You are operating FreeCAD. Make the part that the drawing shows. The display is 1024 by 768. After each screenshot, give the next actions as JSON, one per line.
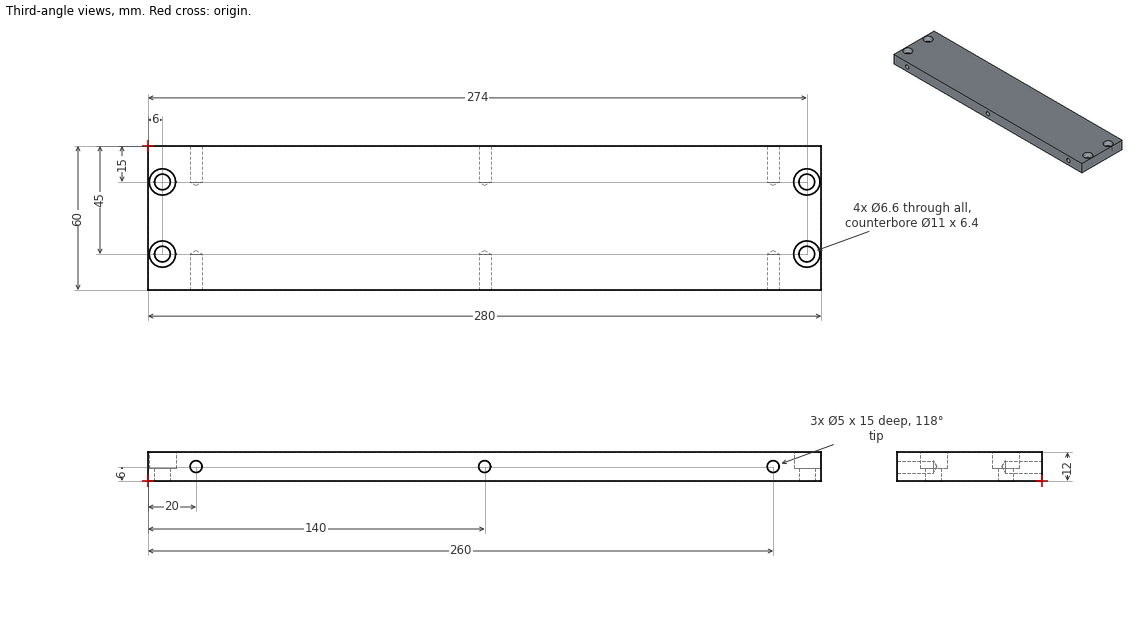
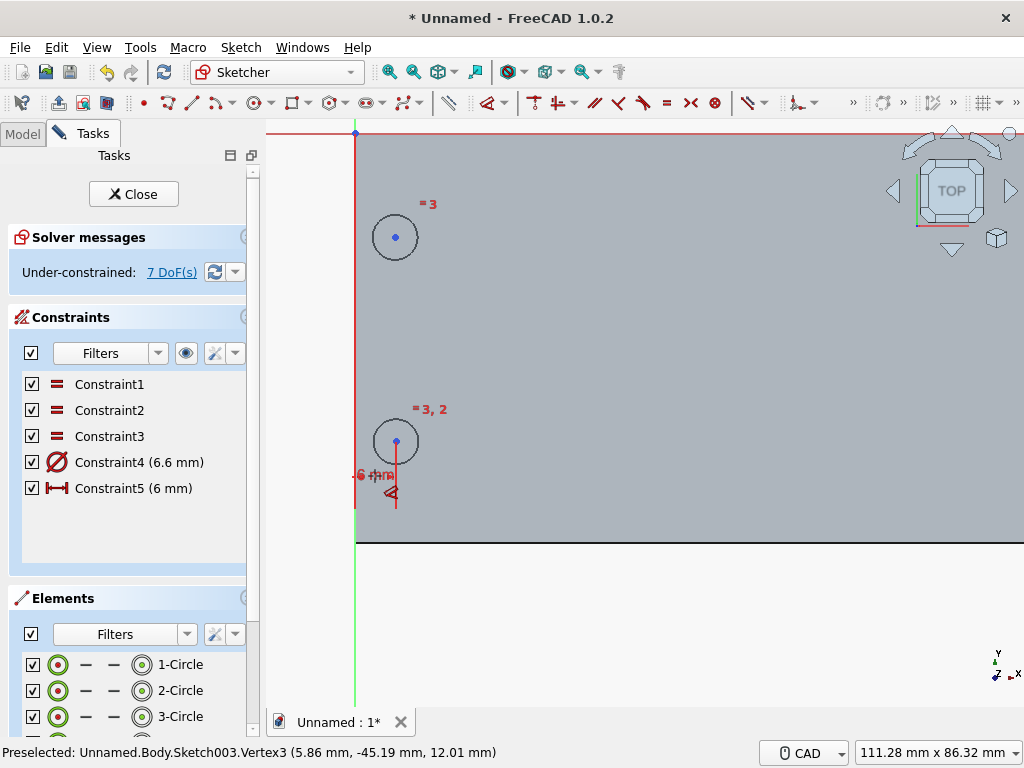
{"action": "left_click", "coordinate": [395, 237]}
{"action": "left_click", "coordinate": [375, 271]}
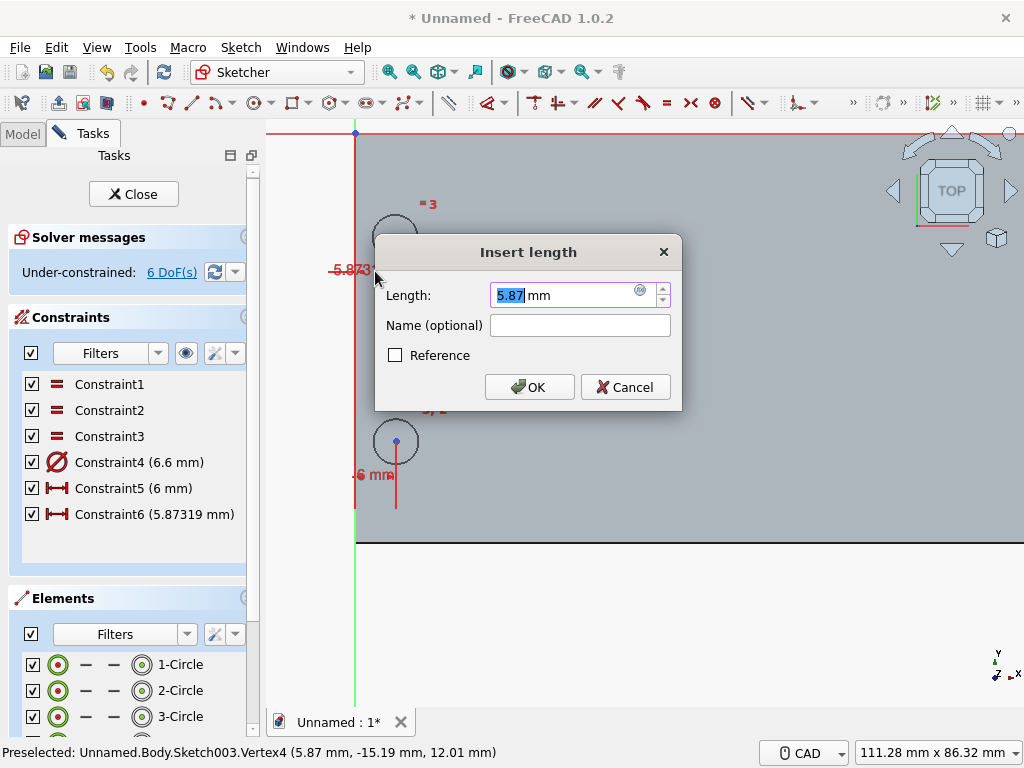
{"action": "type", "text": "6"}
{"action": "key", "text": "Return"}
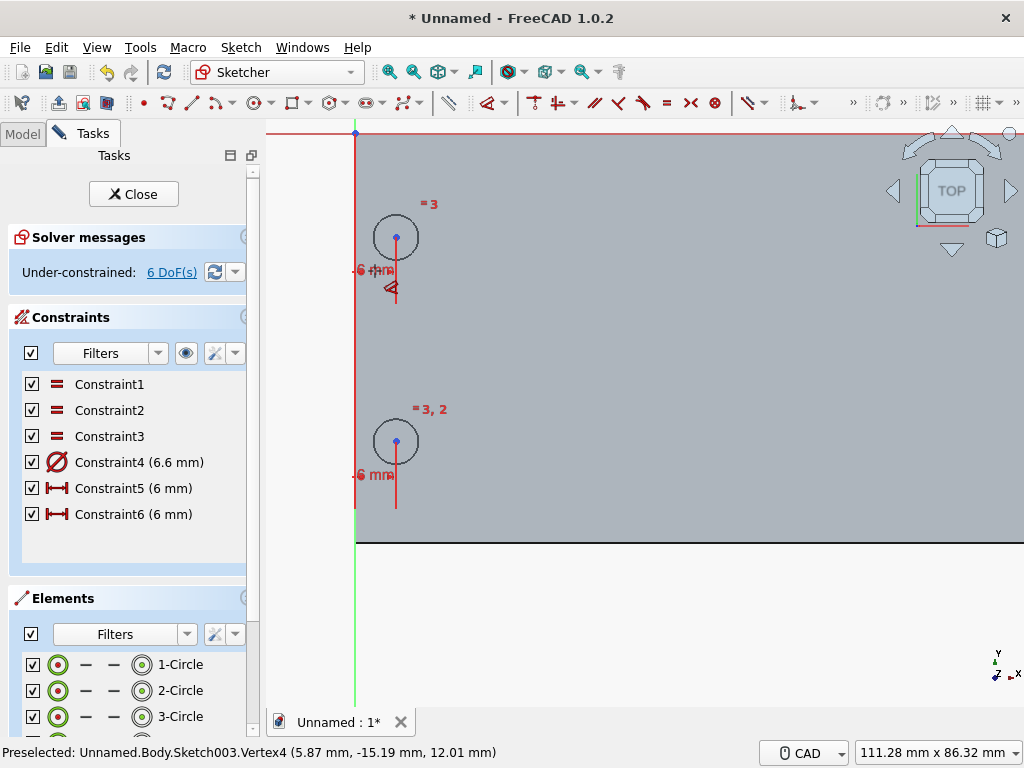
{"action": "scroll", "coordinate": [394, 442], "scroll_direction": "down", "scroll_amount": 8}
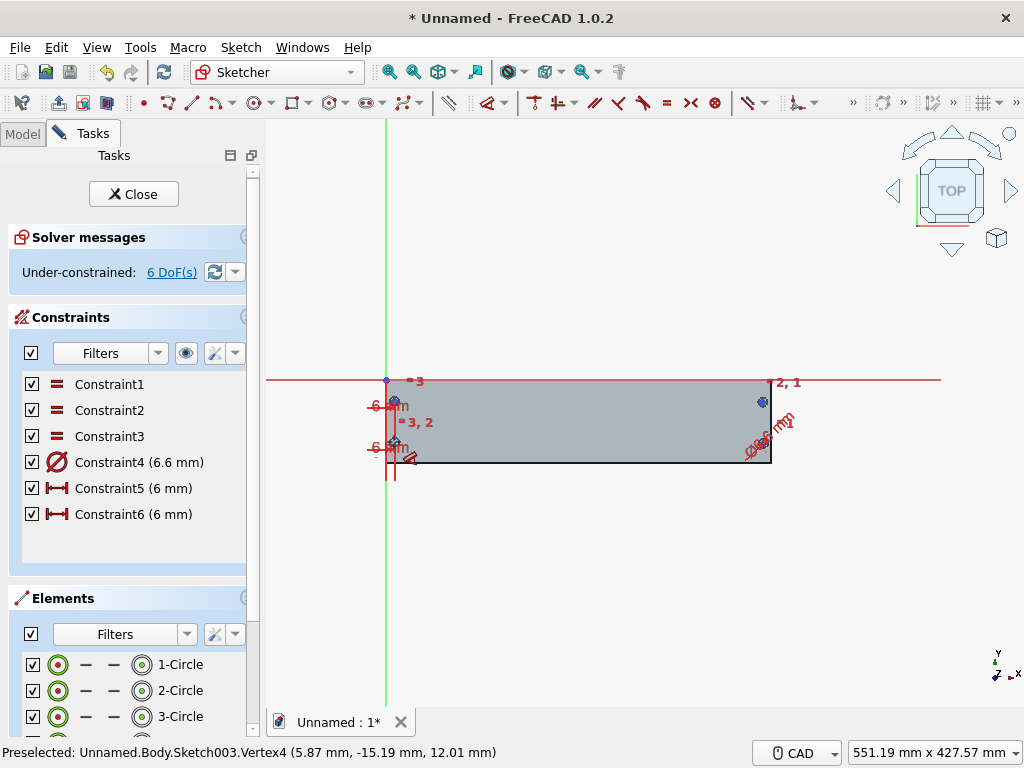
{"action": "left_click", "coordinate": [764, 443]}
{"action": "left_click", "coordinate": [798, 412]}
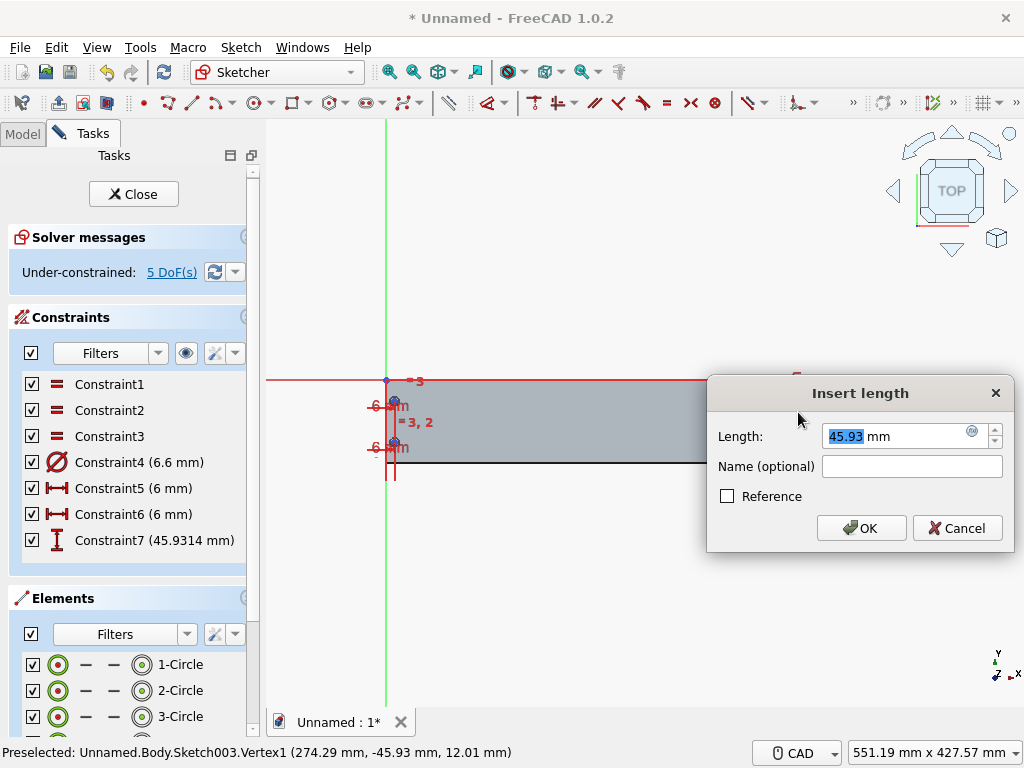
{"action": "type", "text": "45"}
{"action": "key", "text": "Return"}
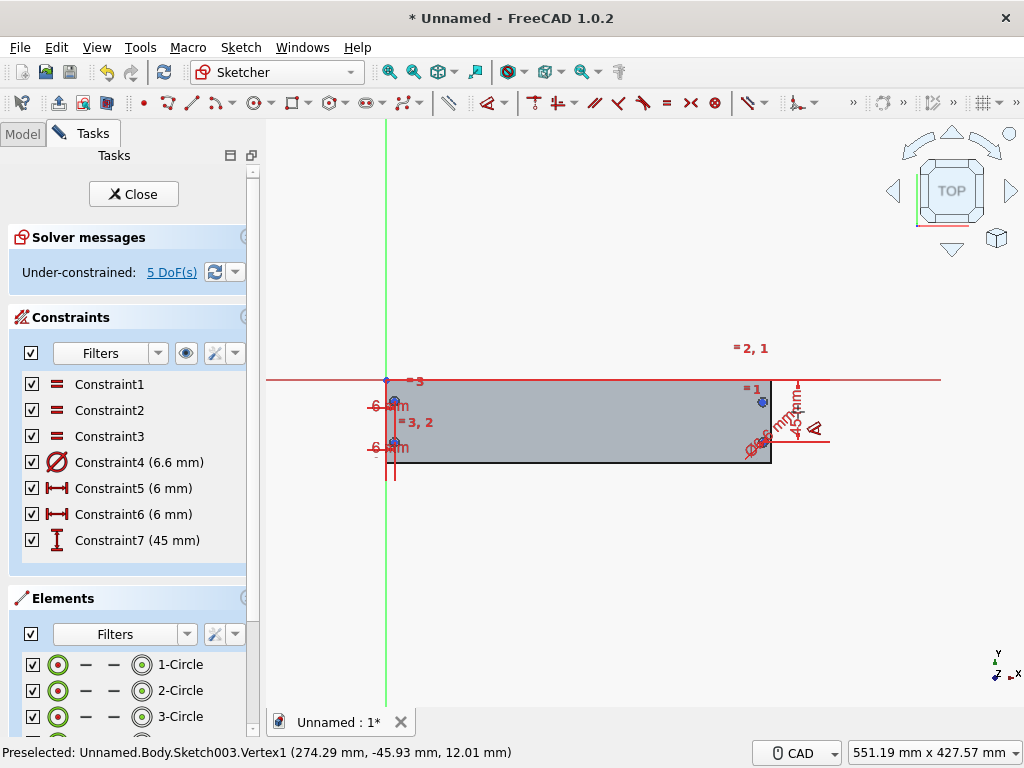
{"action": "scroll", "coordinate": [763, 402], "scroll_direction": "up", "scroll_amount": 4}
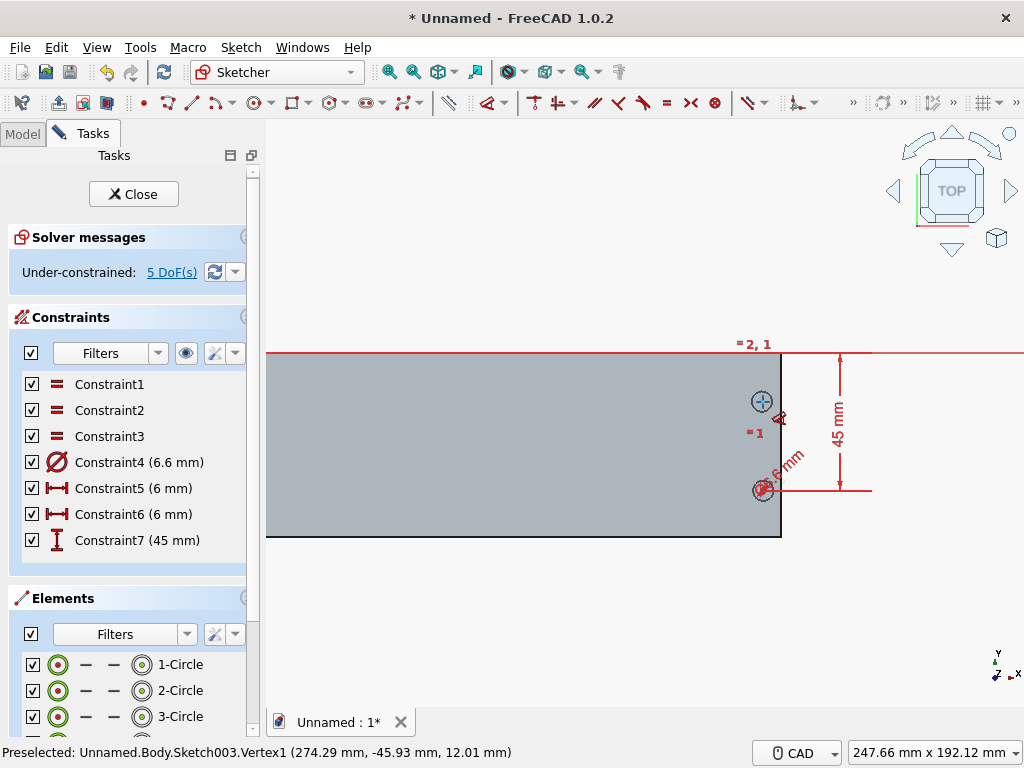
{"action": "left_click", "coordinate": [762, 402]}
{"action": "left_click", "coordinate": [796, 377]}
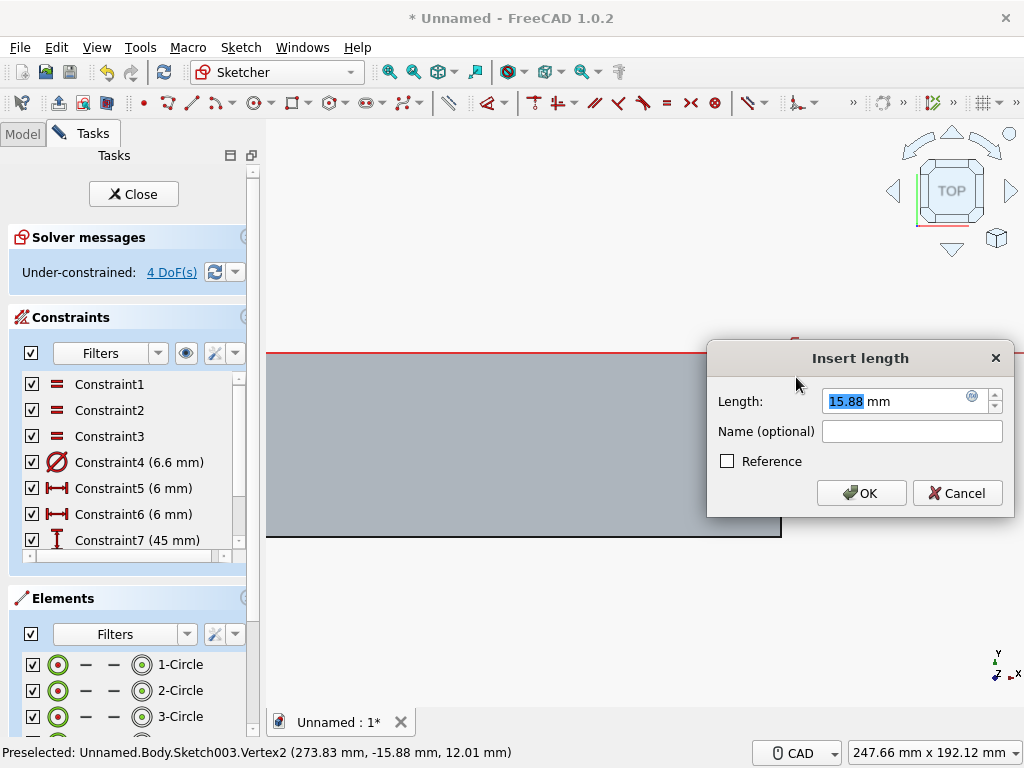
{"action": "type", "text": "15"}
{"action": "key", "text": "Return"}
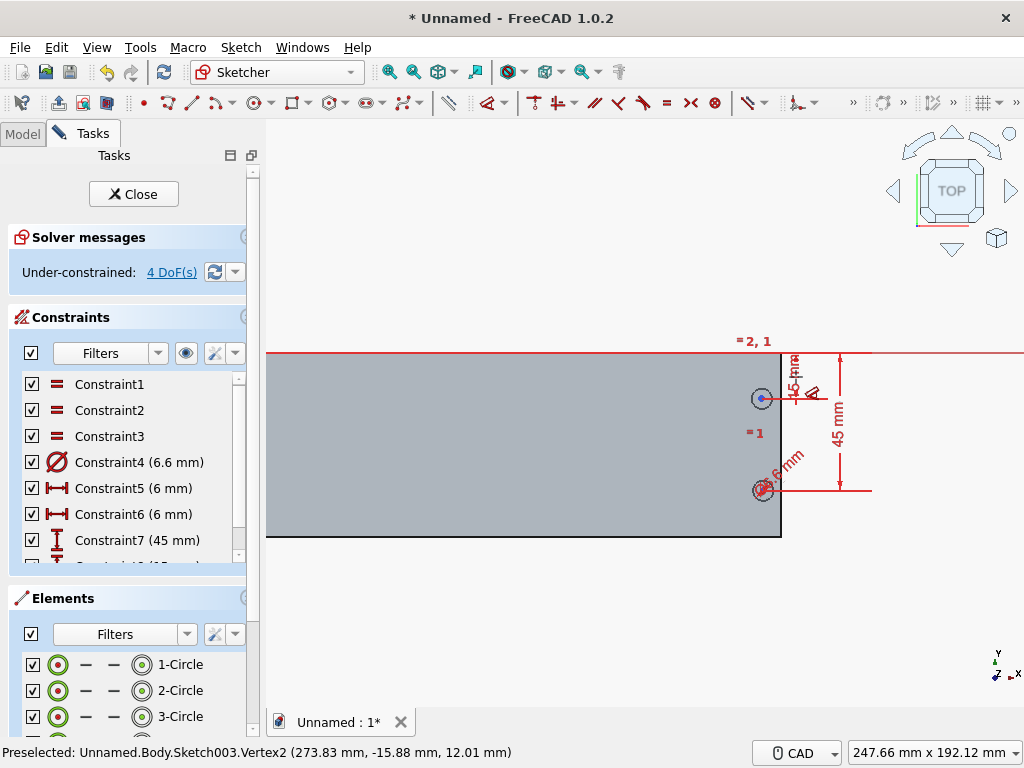
{"action": "scroll", "coordinate": [763, 402], "scroll_direction": "down", "scroll_amount": 4}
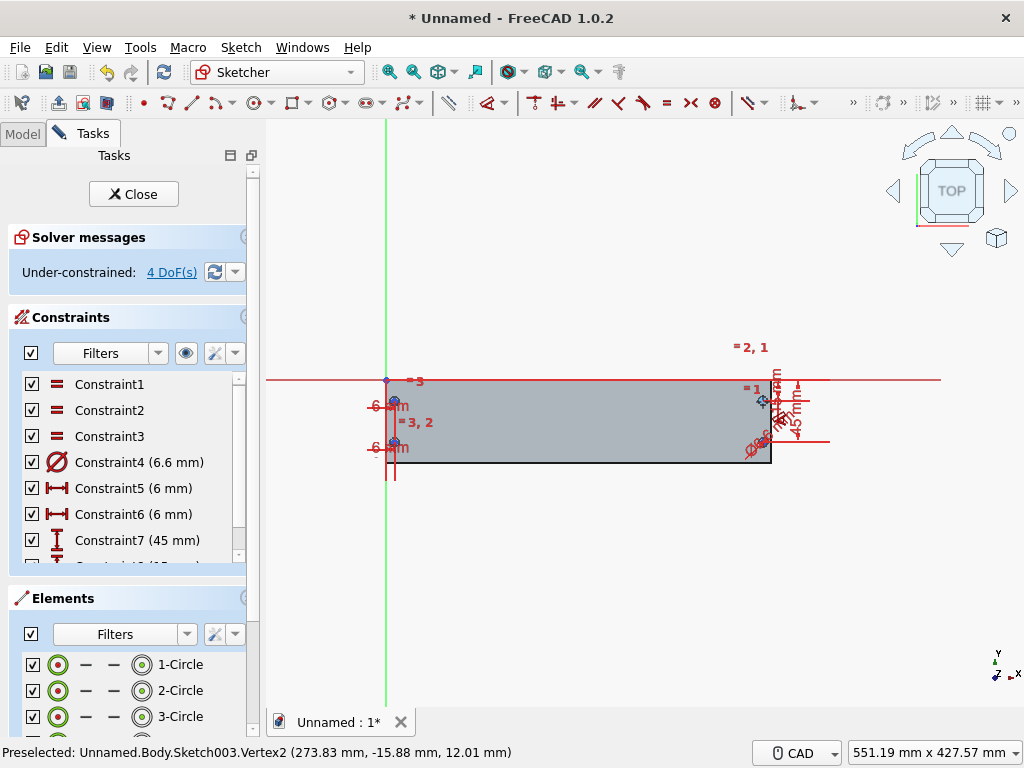
{"action": "left_click", "coordinate": [395, 442]}
{"action": "left_click", "coordinate": [304, 411]}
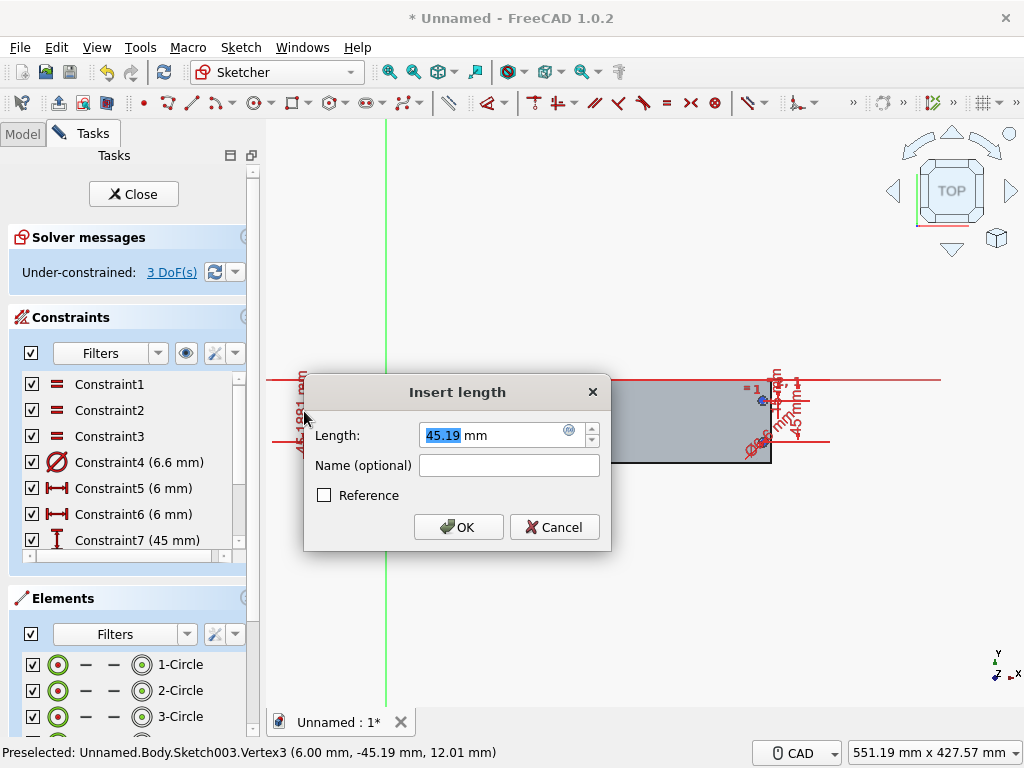
{"action": "type", "text": "45"}
{"action": "key", "text": "Return"}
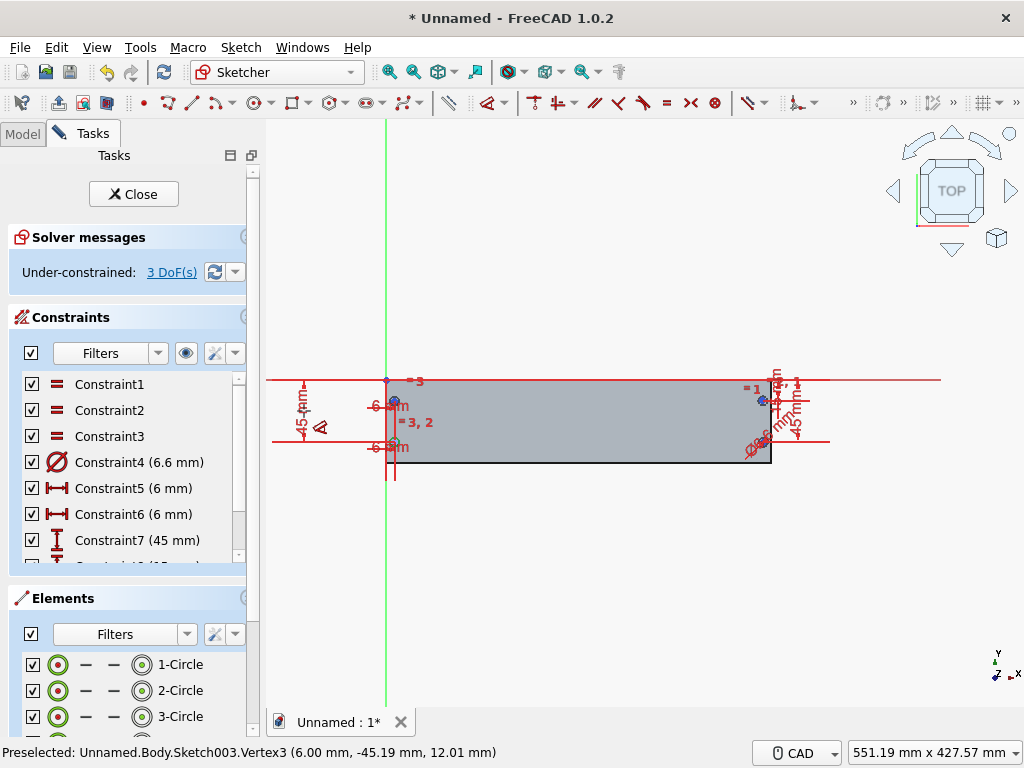
{"action": "scroll", "coordinate": [395, 401], "scroll_direction": "up", "scroll_amount": 4}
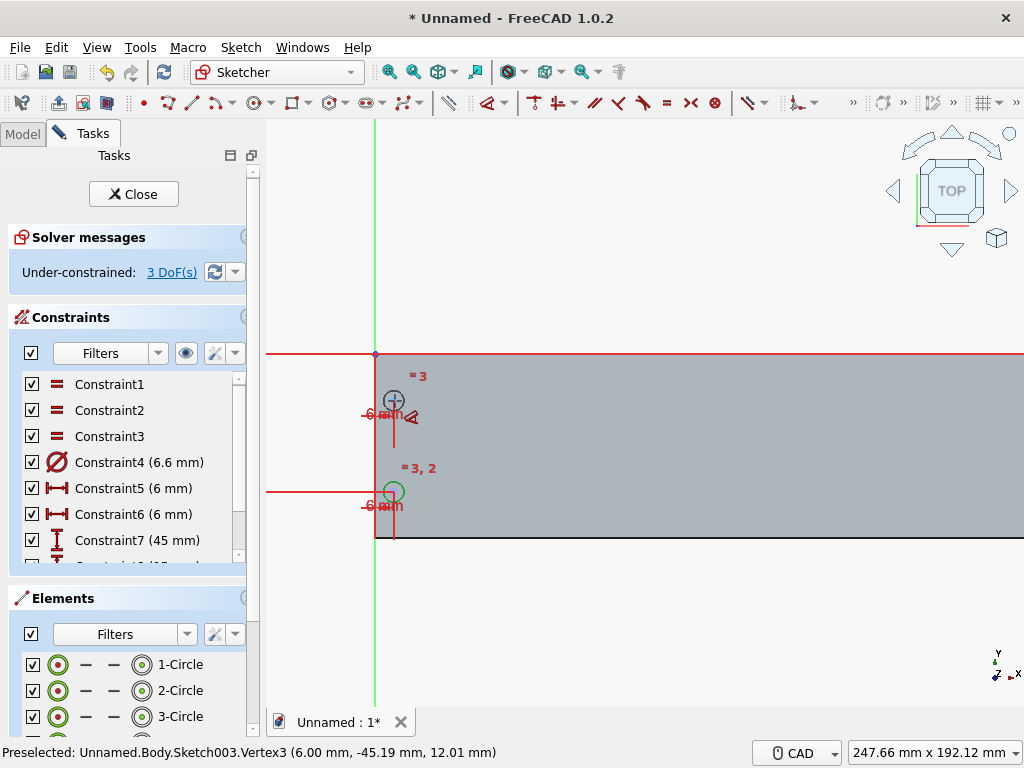
{"action": "left_click", "coordinate": [394, 401]}
{"action": "left_click", "coordinate": [341, 377]}